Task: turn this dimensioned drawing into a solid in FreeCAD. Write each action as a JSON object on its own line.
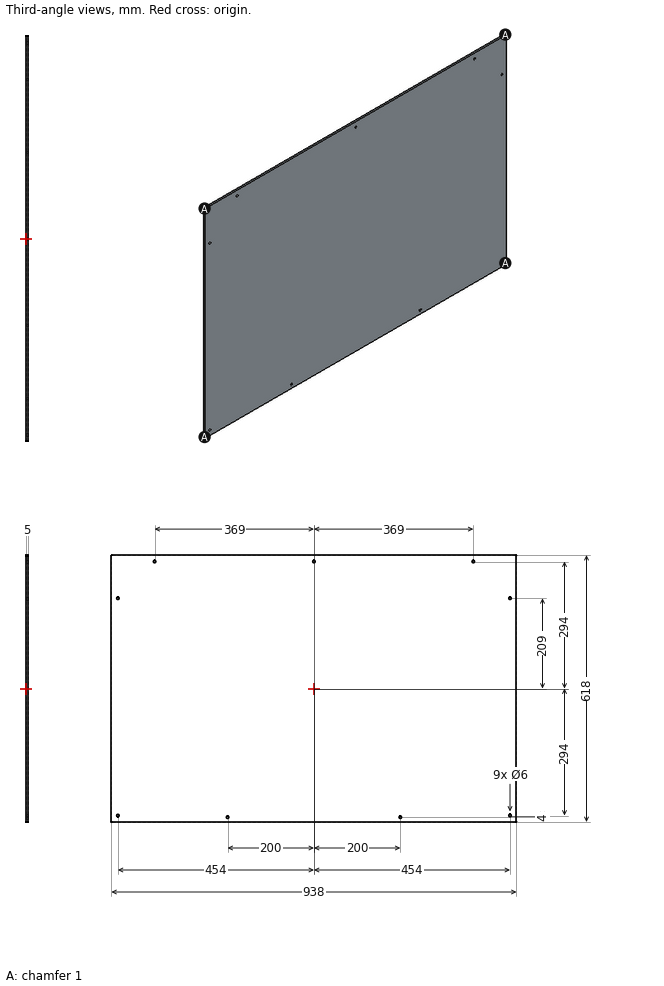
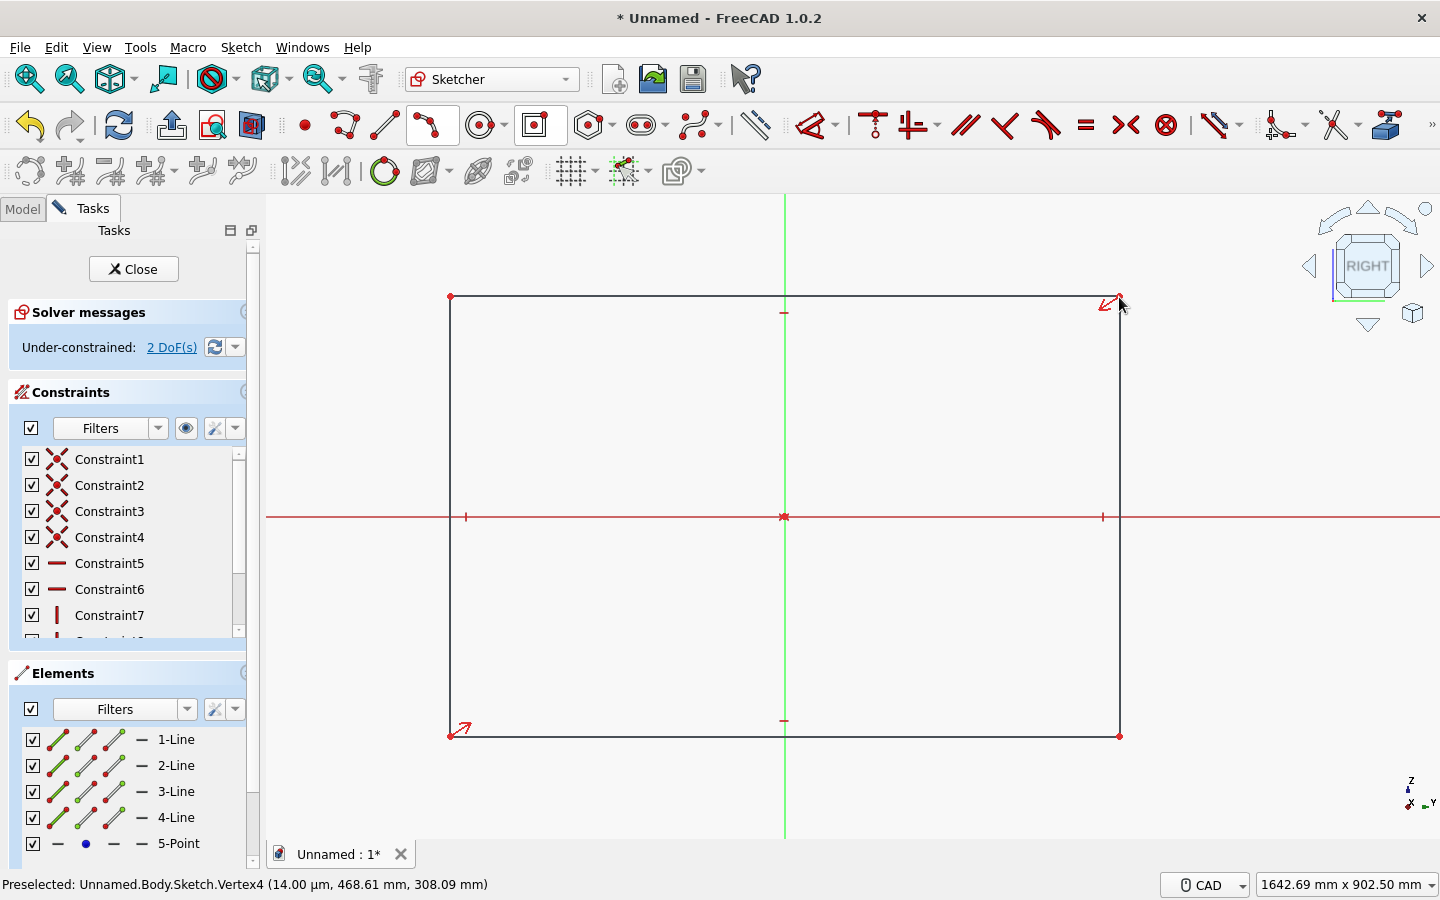
{"action": "left_click", "coordinate": [810, 126]}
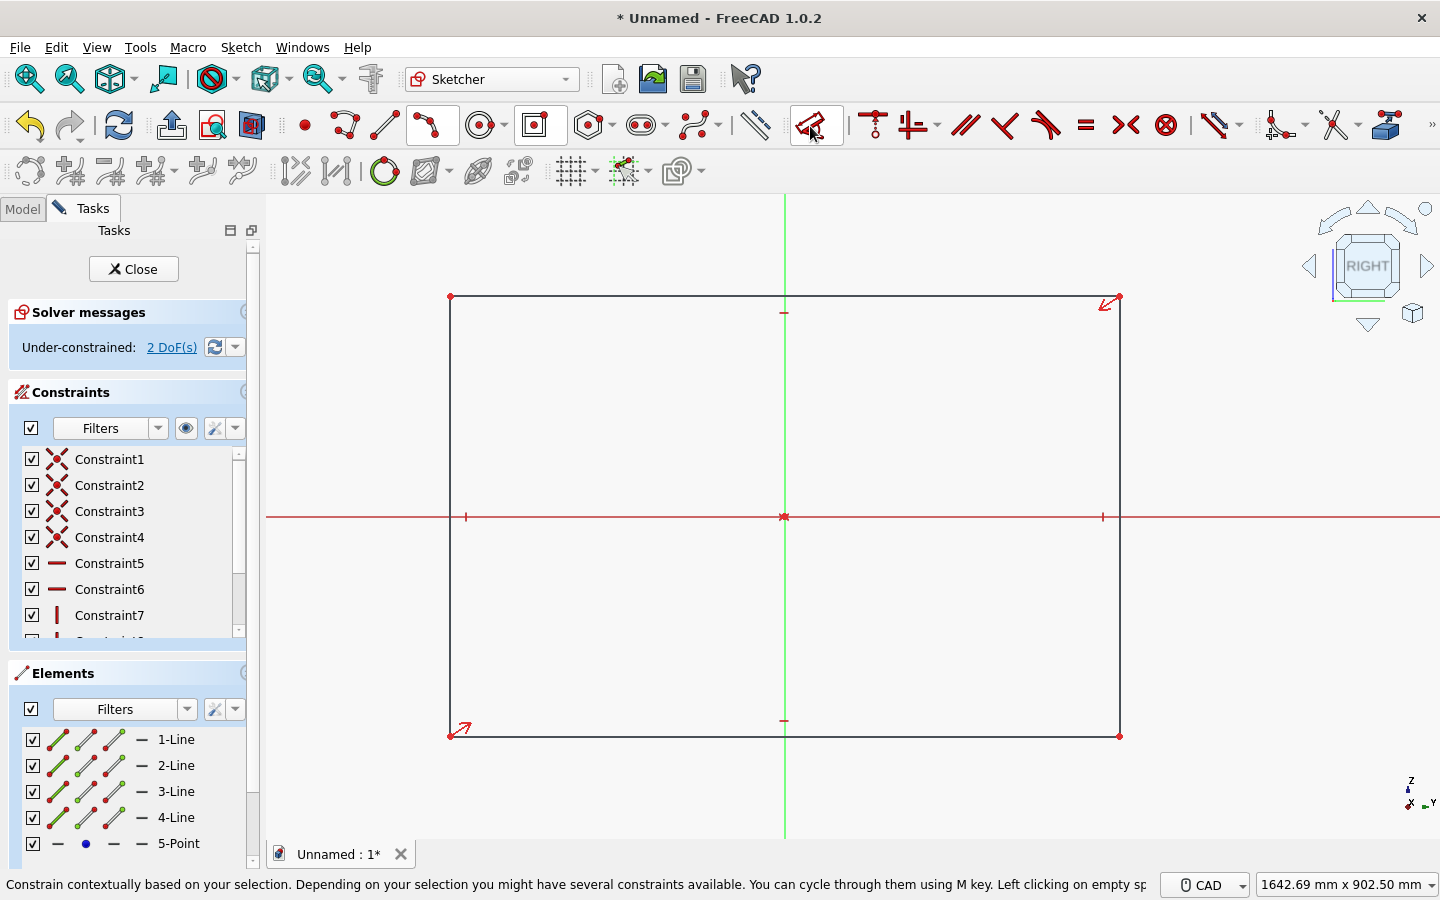
{"action": "left_click", "coordinate": [651, 737]}
{"action": "left_click", "coordinate": [631, 771]}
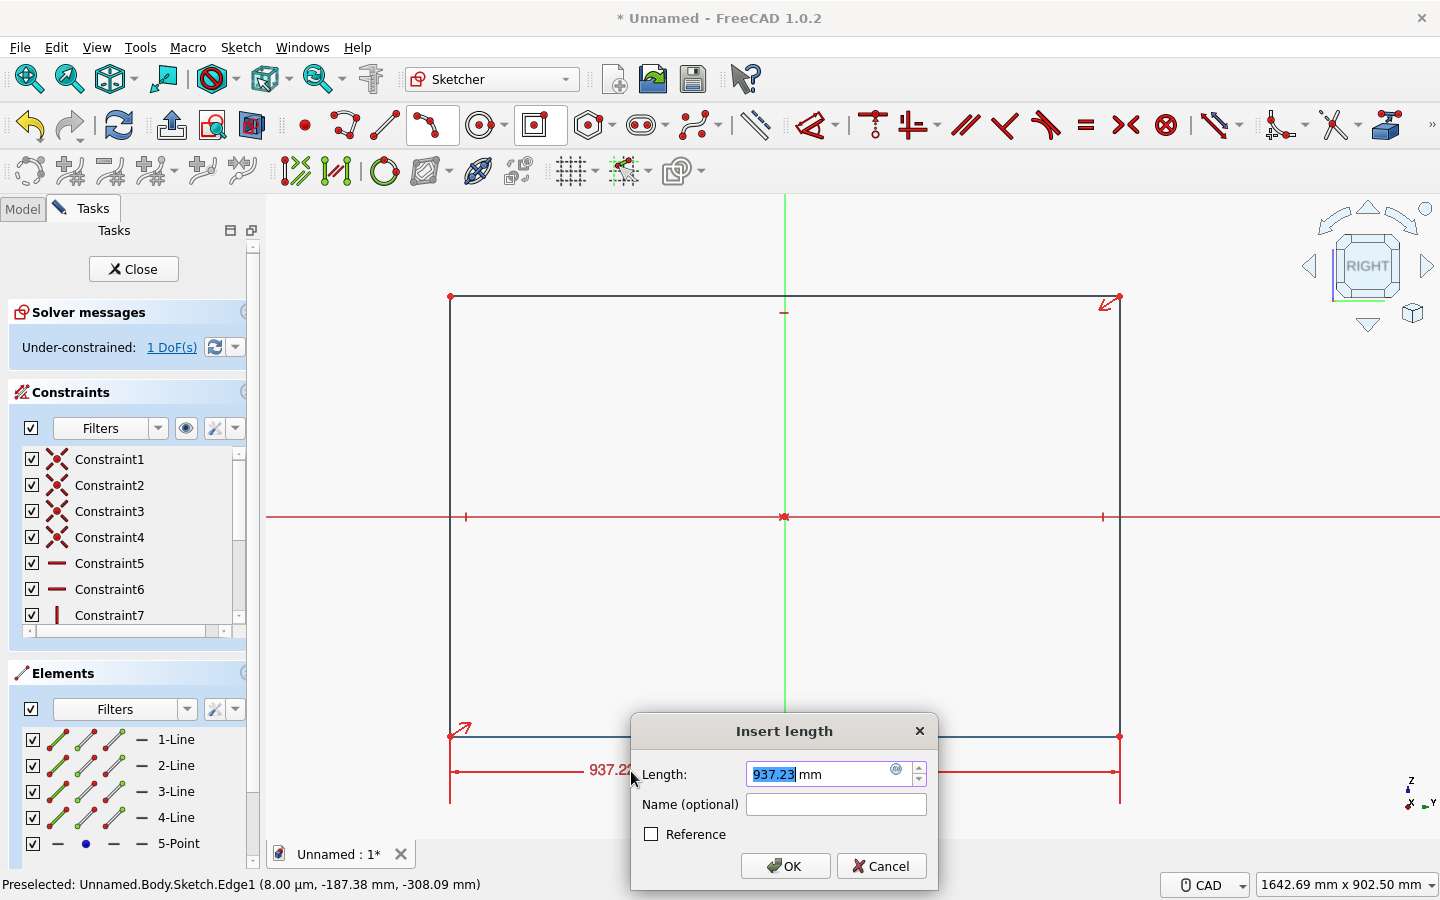
{"action": "type", "text": "938"}
{"action": "key", "text": "Return"}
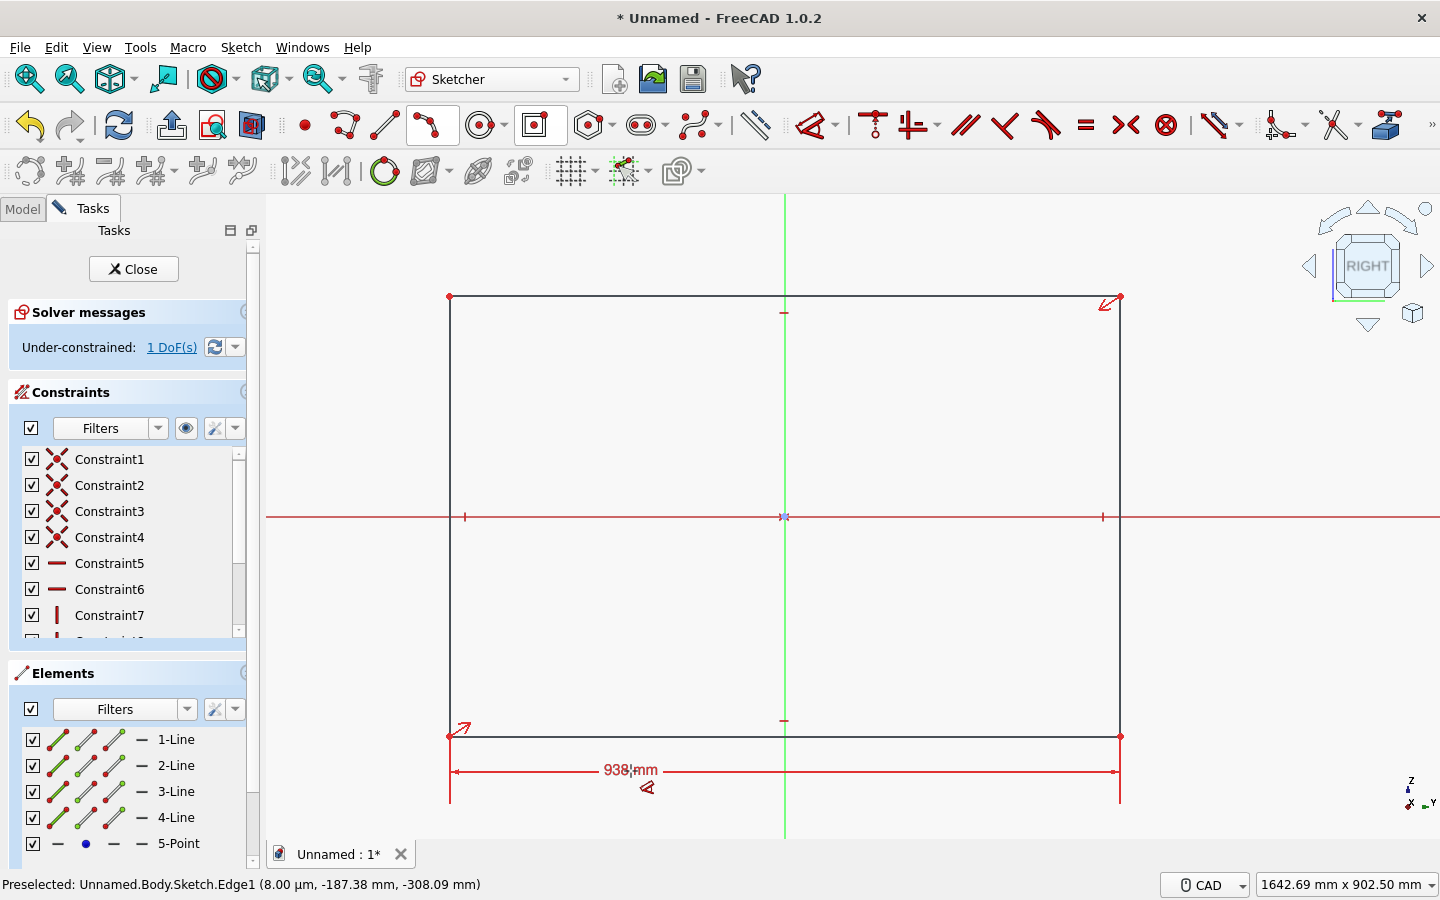
{"action": "left_click", "coordinate": [1120, 605]}
{"action": "left_click", "coordinate": [1154, 415]}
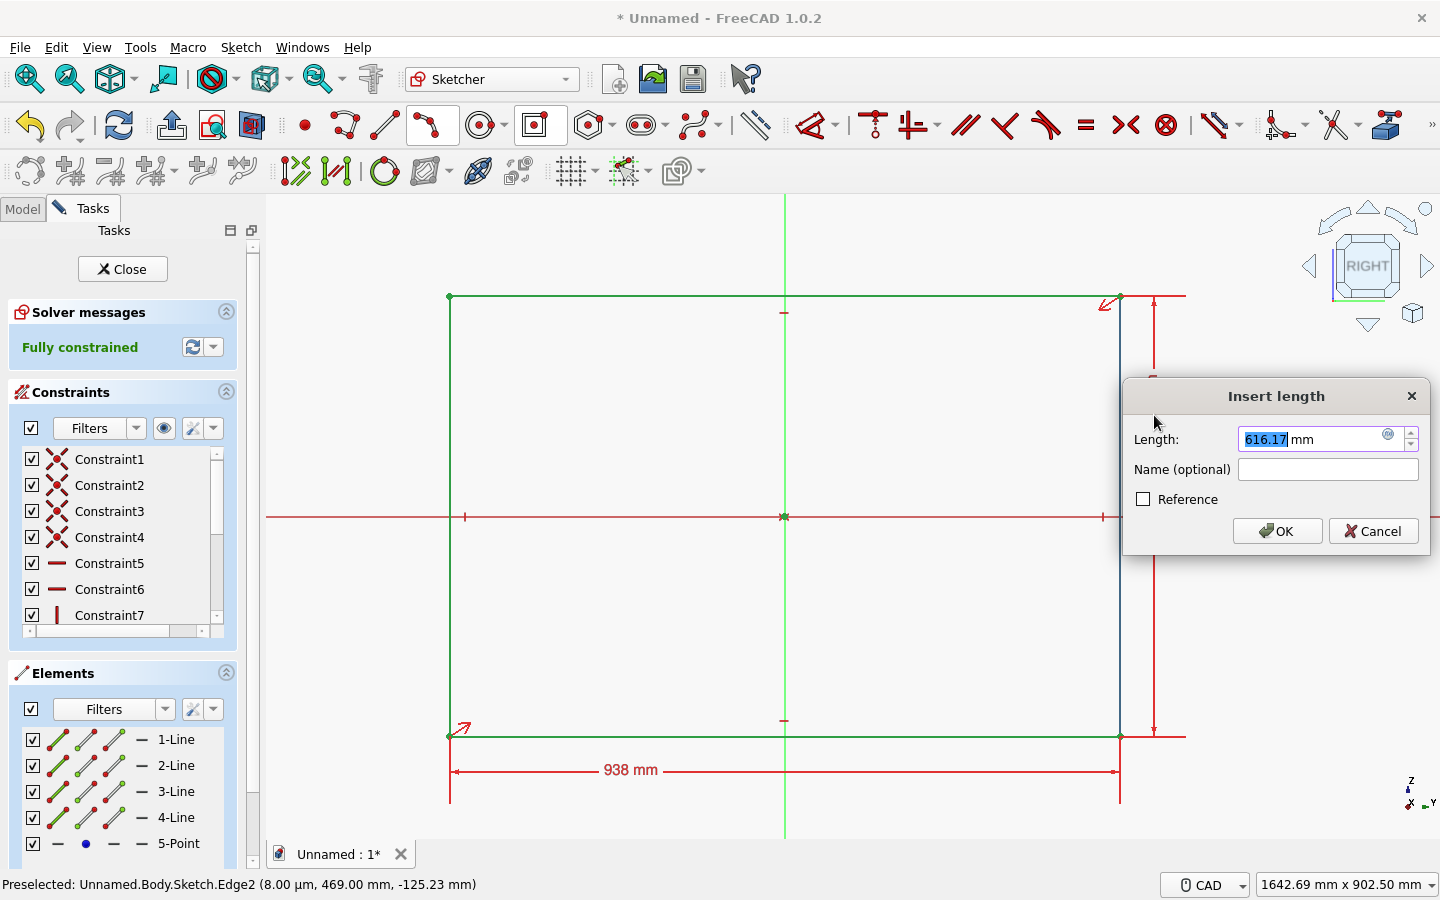
{"action": "type", "text": "618"}
{"action": "key", "text": "Return"}
{"action": "key", "text": "Escape"}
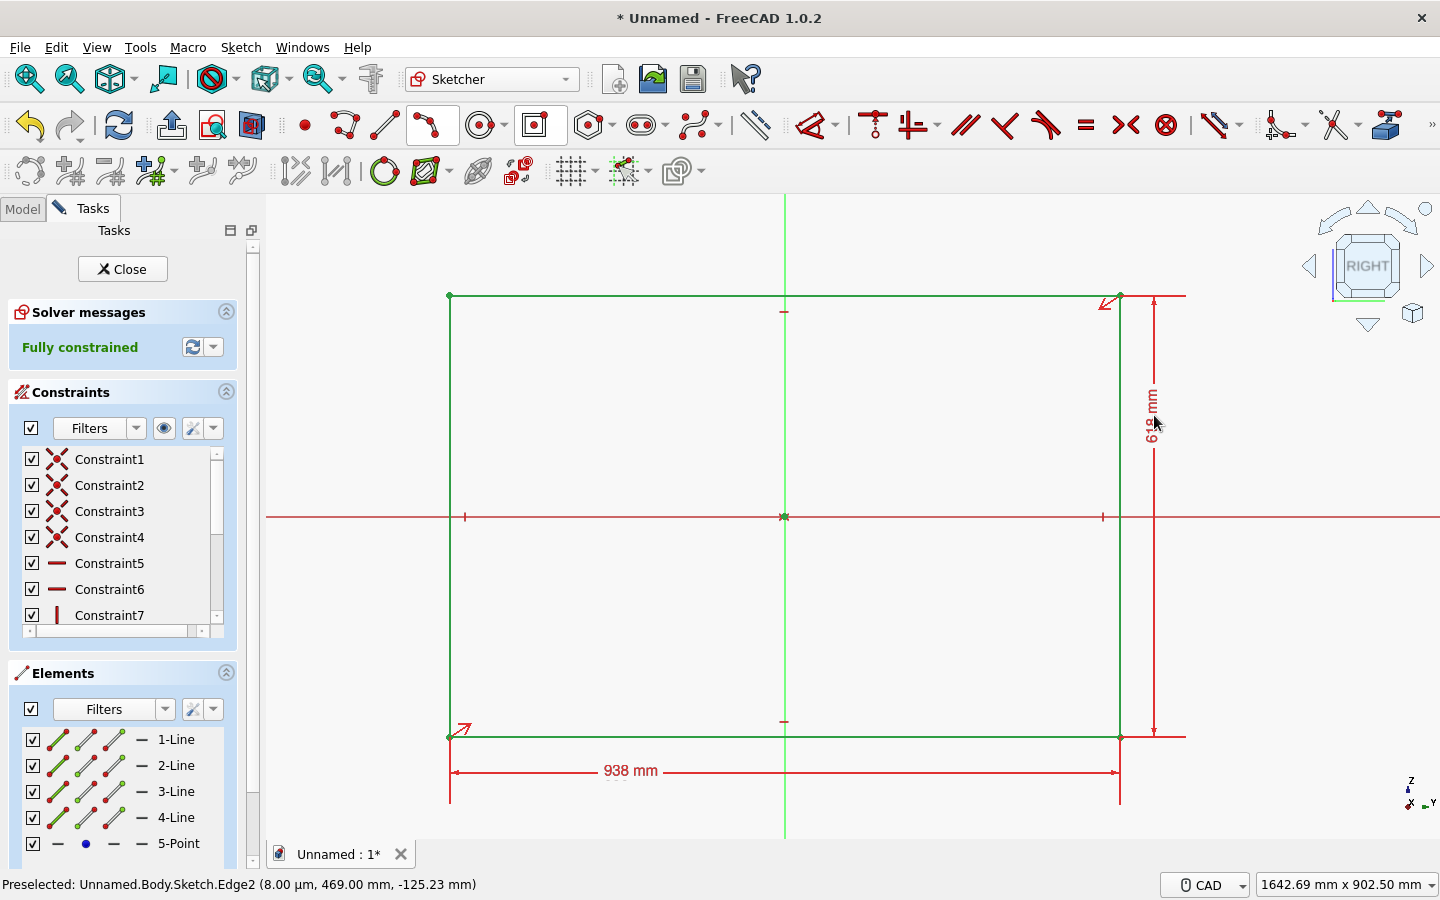
{"action": "left_click", "coordinate": [123, 269]}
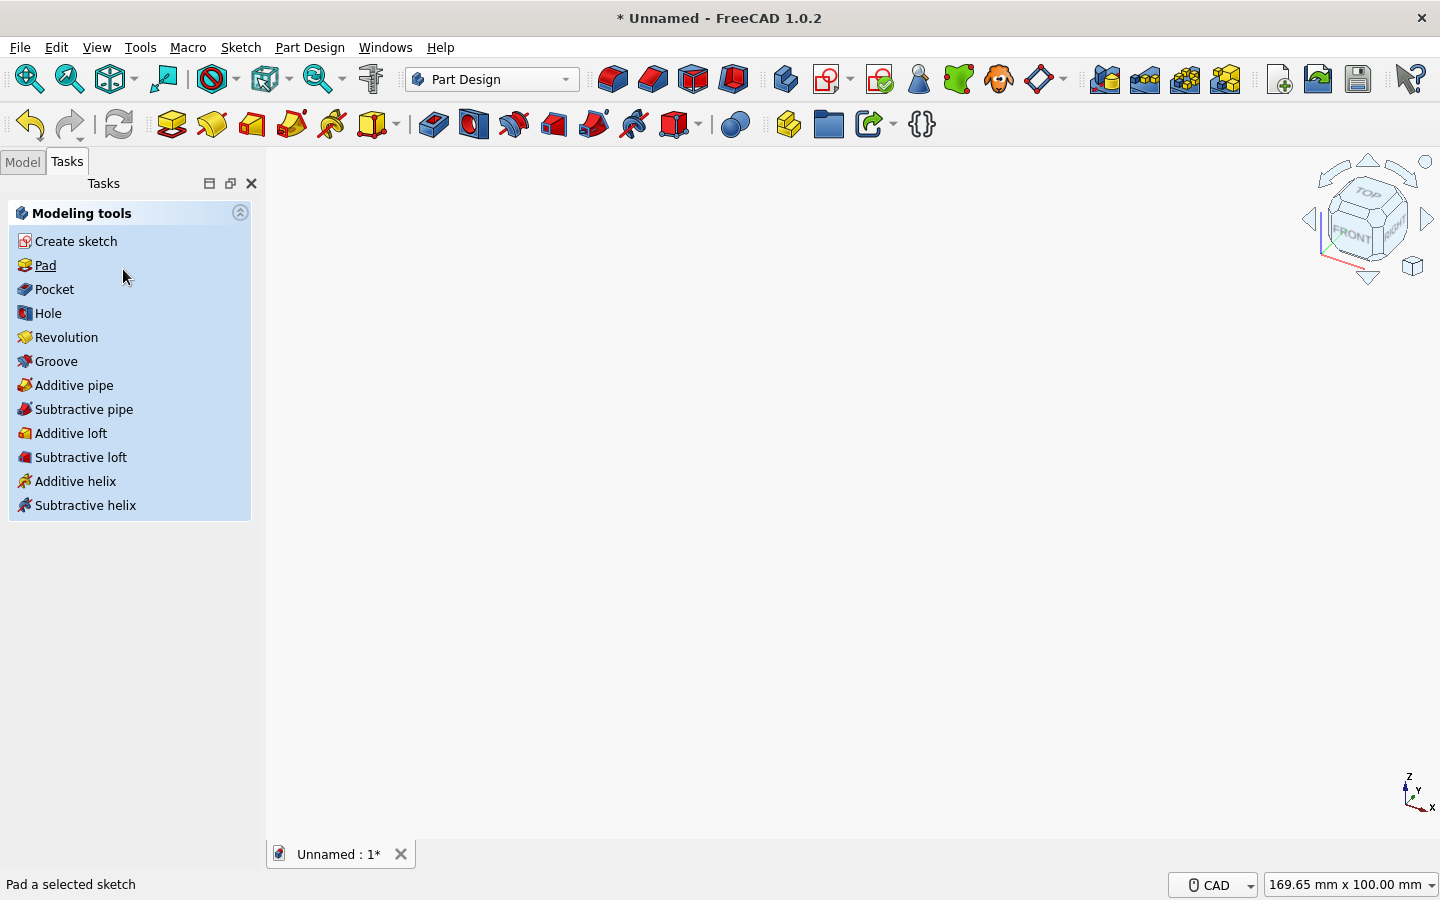
{"action": "left_click", "coordinate": [172, 124]}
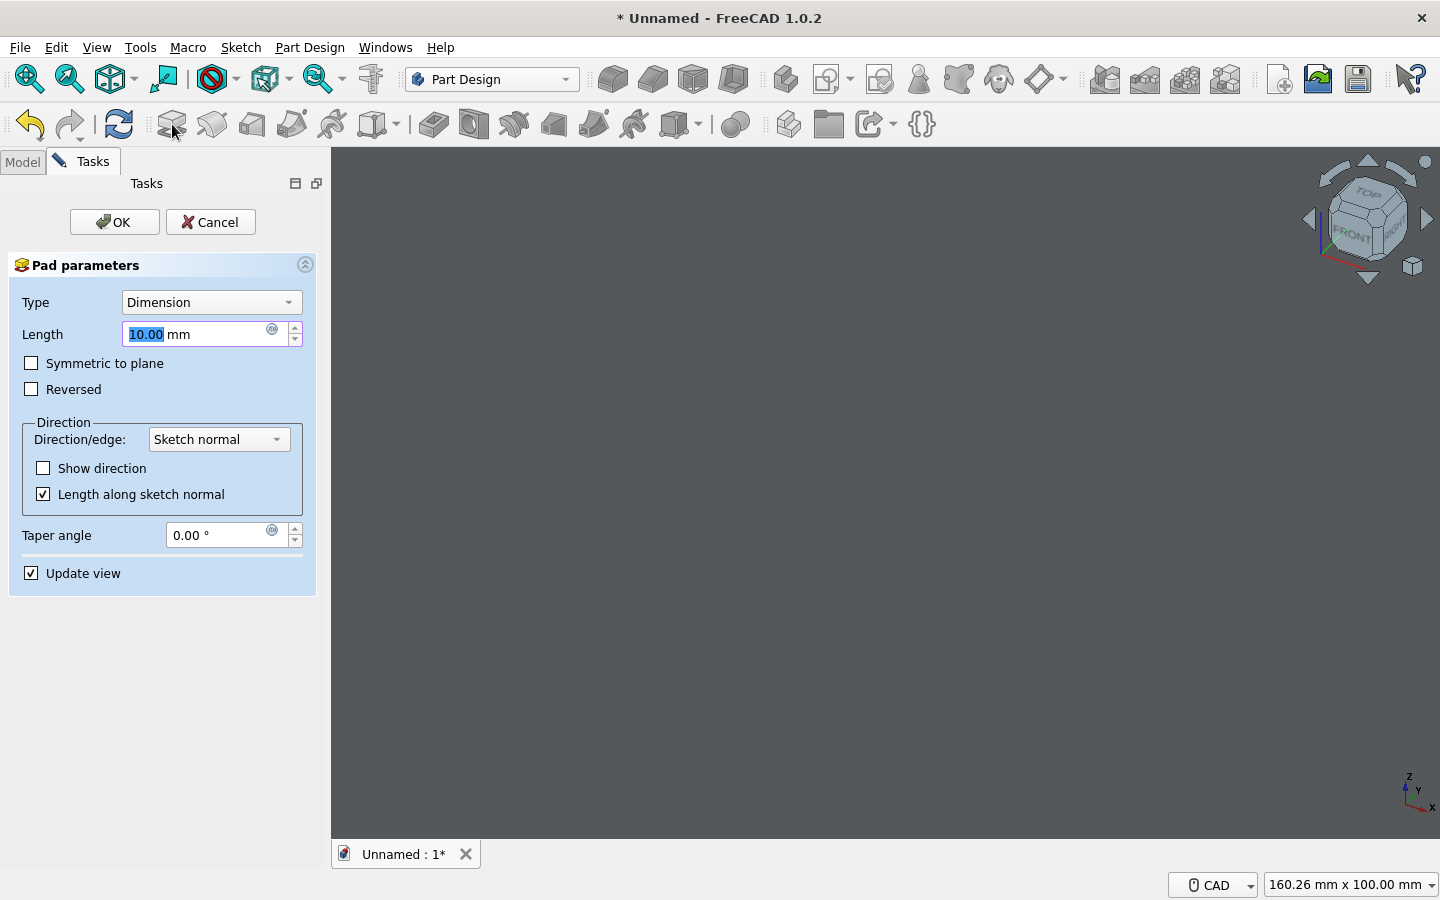
{"action": "type", "text": "5"}
{"action": "key", "text": "Tab"}